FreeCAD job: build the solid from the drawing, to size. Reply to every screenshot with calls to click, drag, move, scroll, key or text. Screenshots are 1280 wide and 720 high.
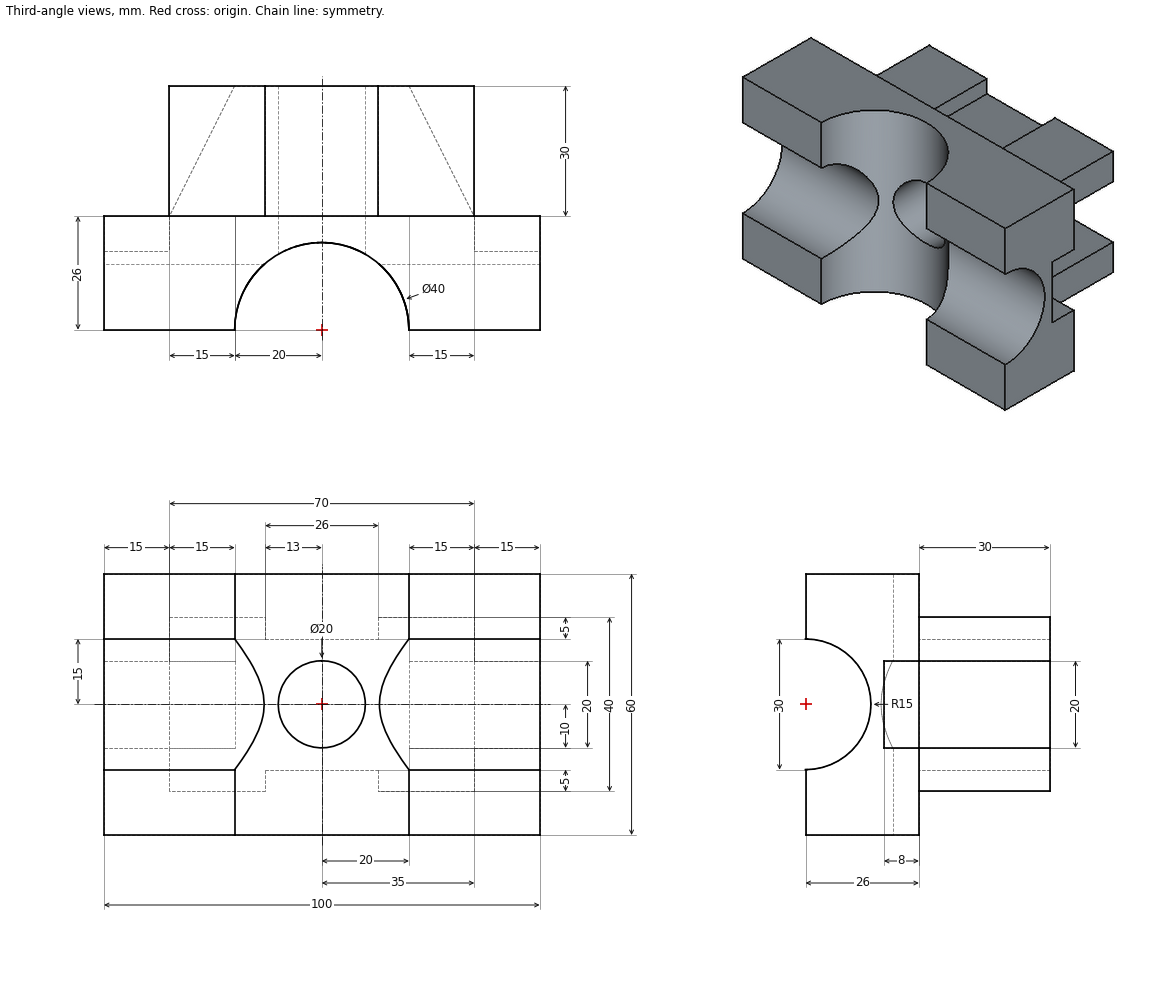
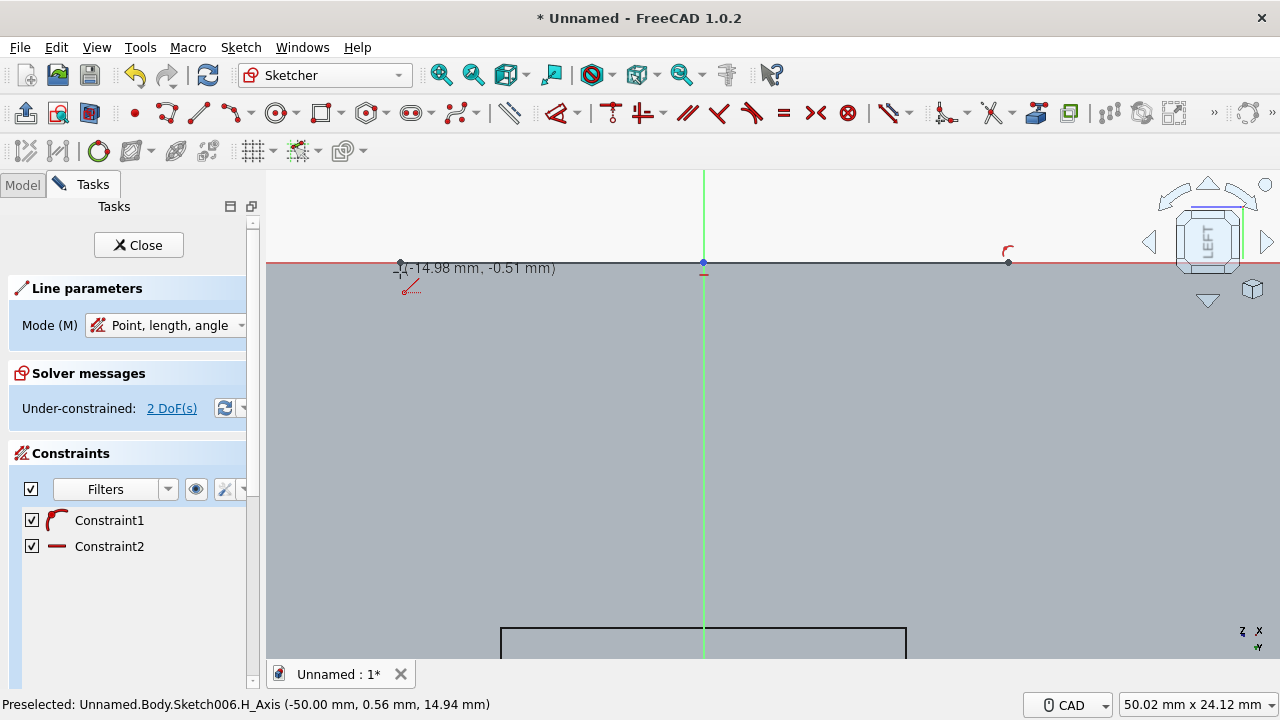
key(g)
key(3)
key(a)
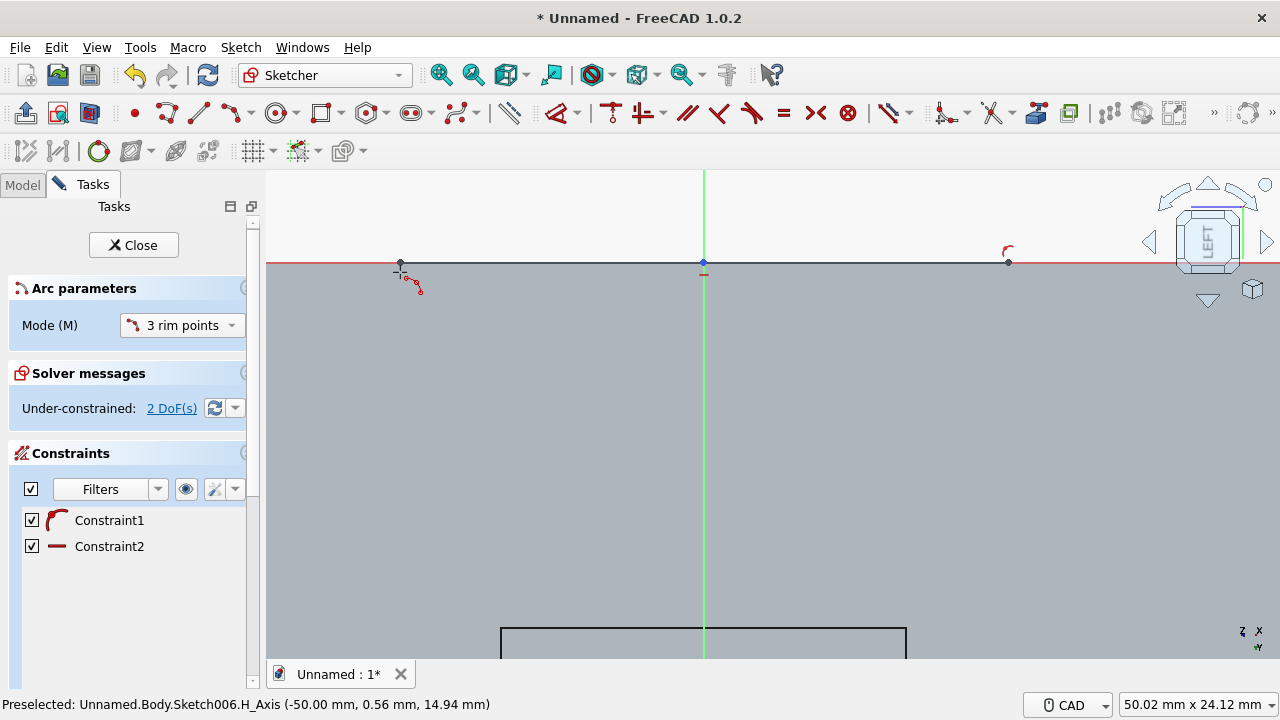
click(400, 272)
click(1008, 263)
click(610, 552)
key(Escape)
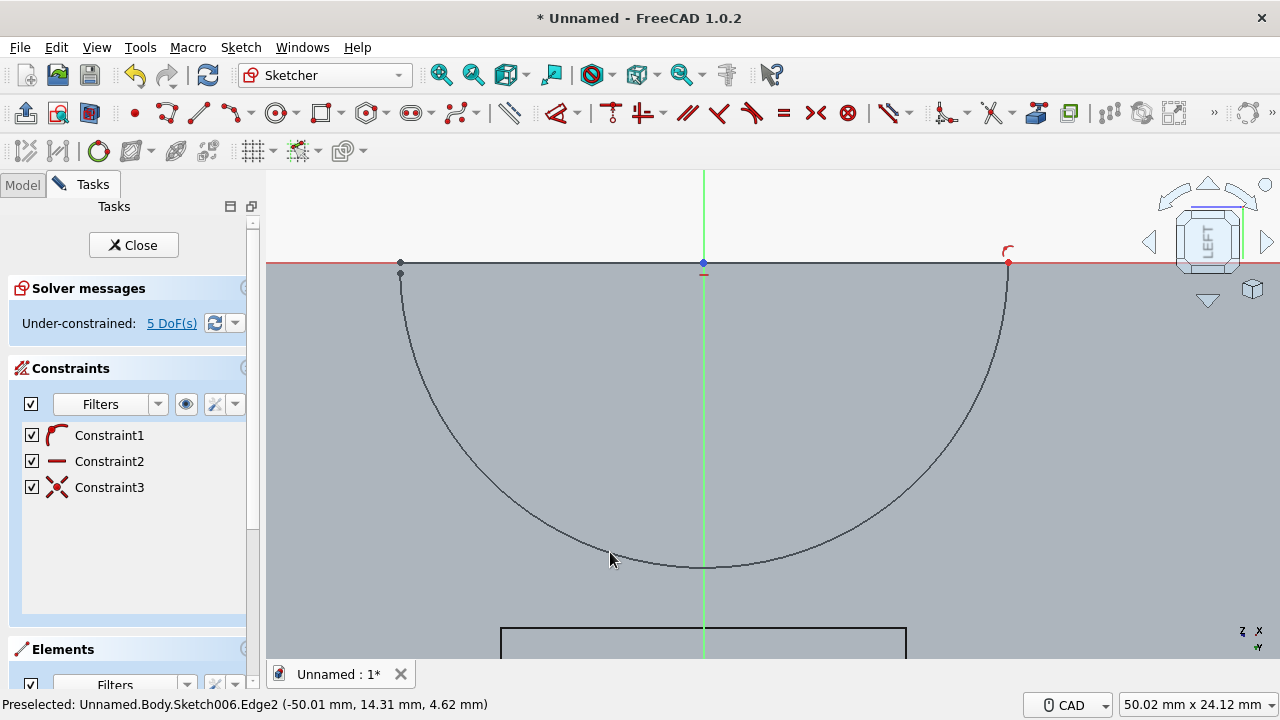
drag(694, 253, 714, 274)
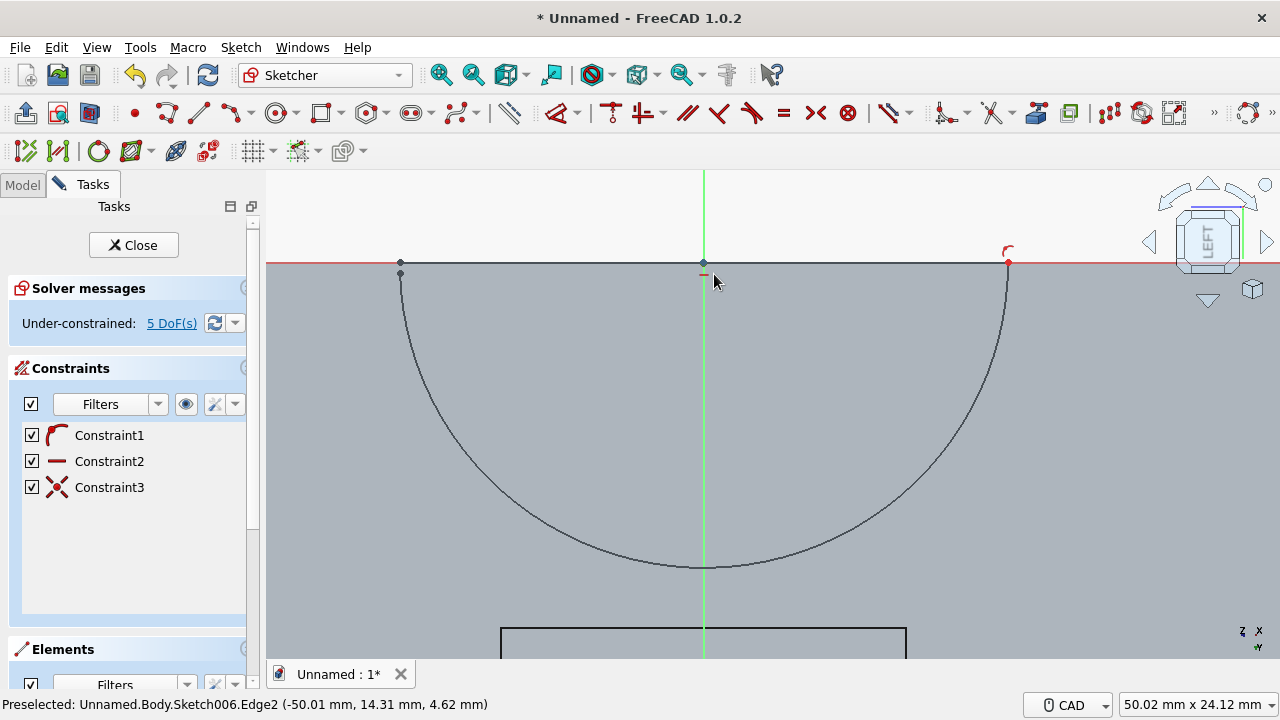
key(c)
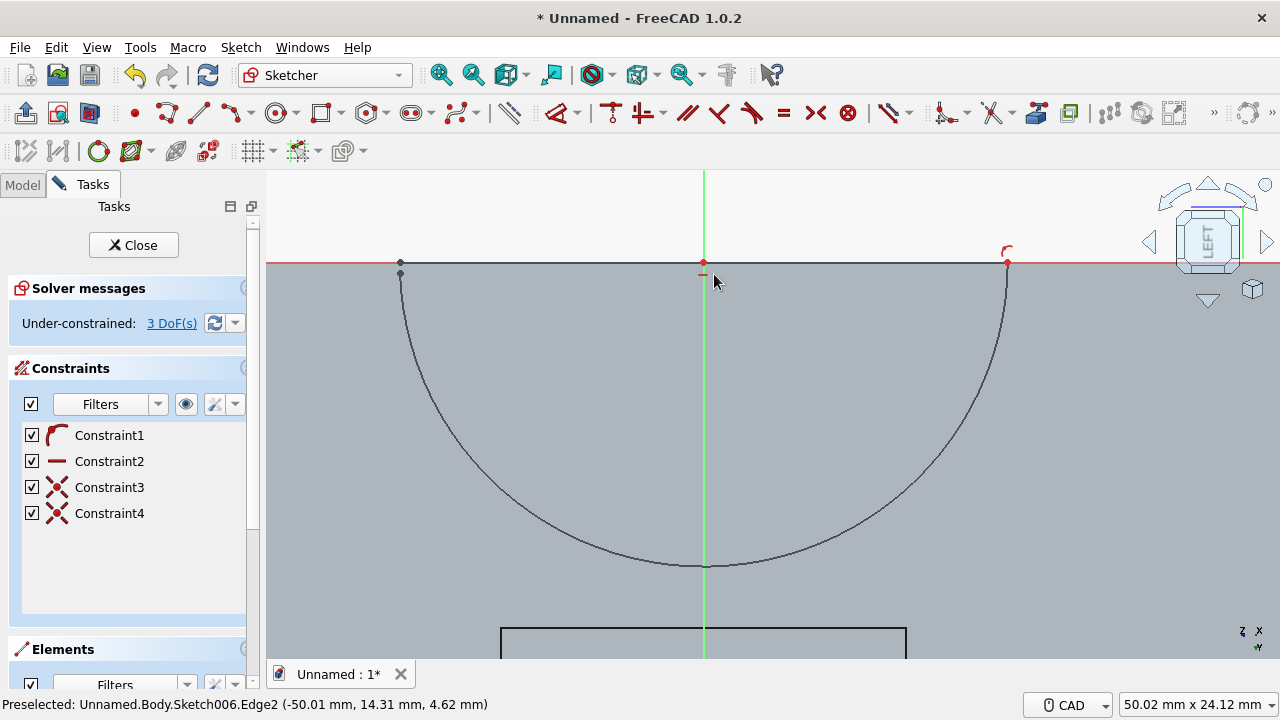
click(556, 114)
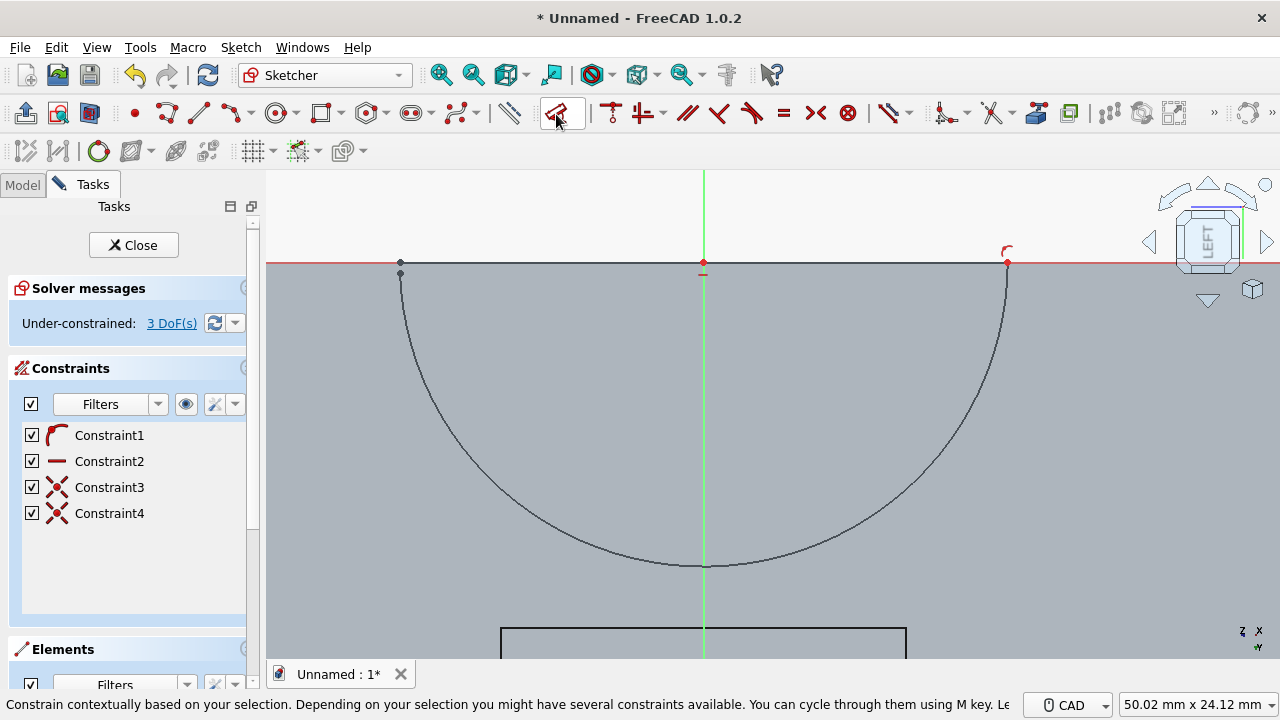
click(531, 513)
click(513, 539)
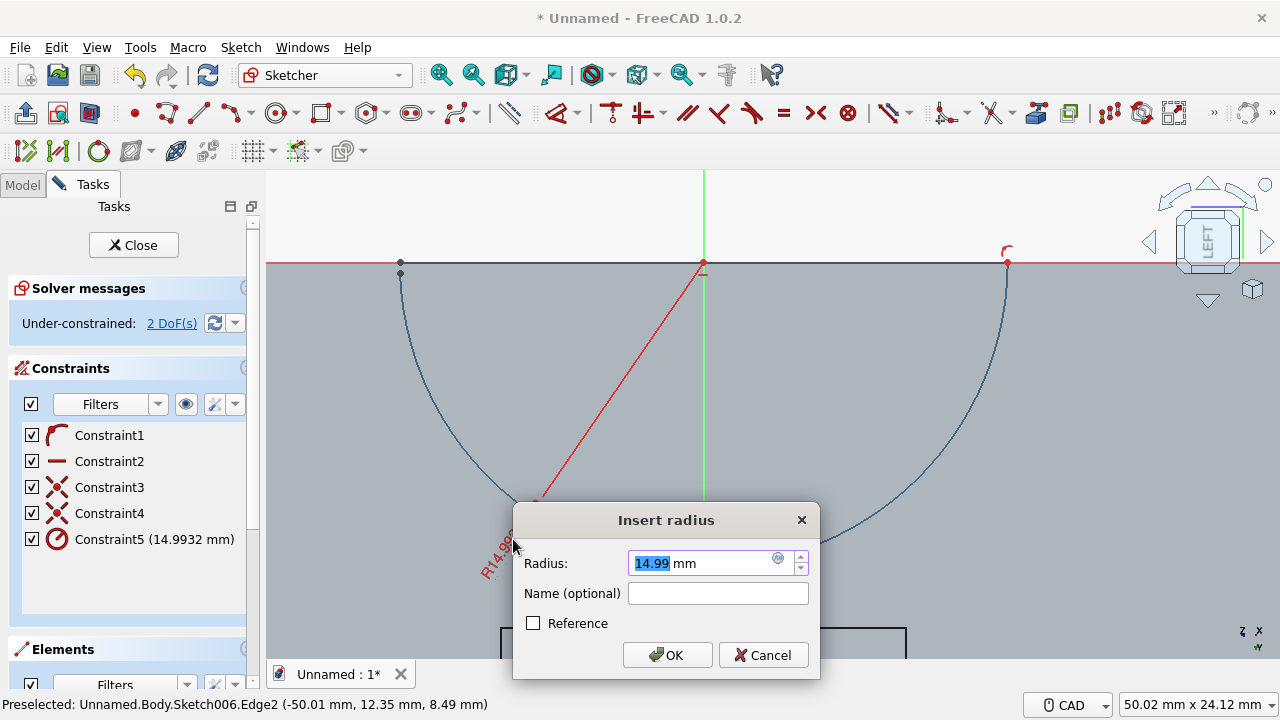
text(15)
key(Return)
key(Escape)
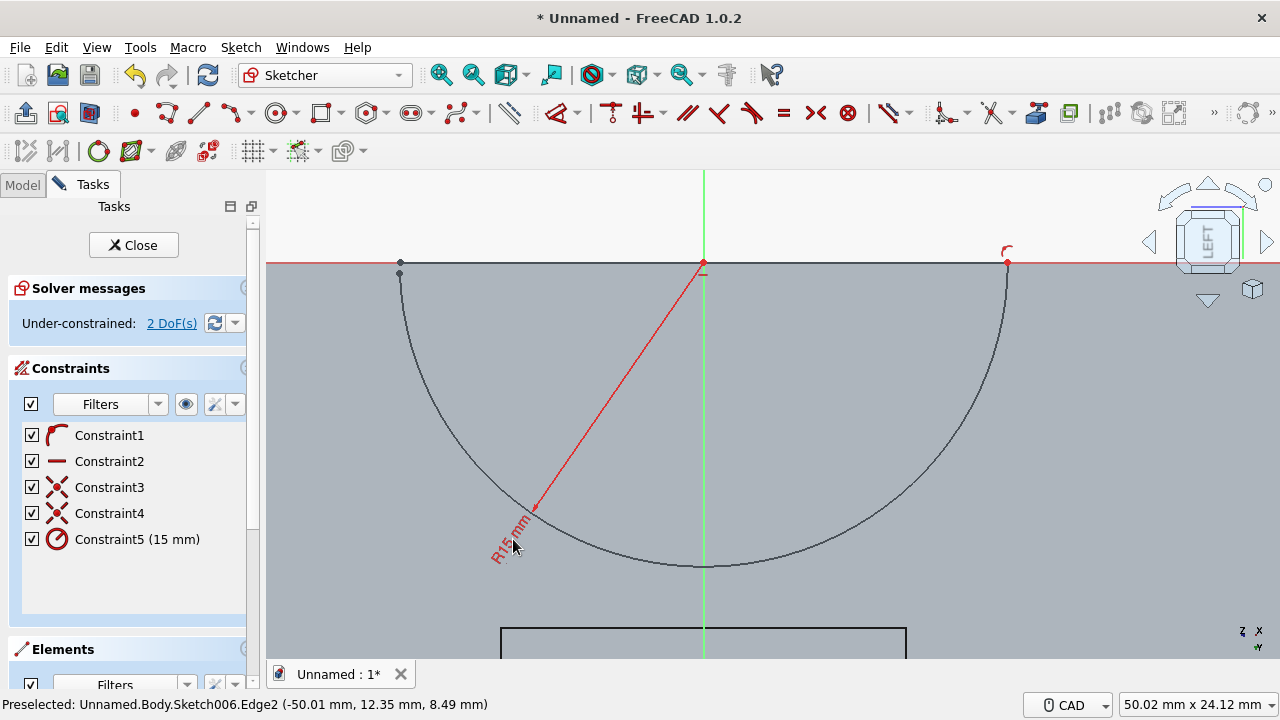
click(400, 273)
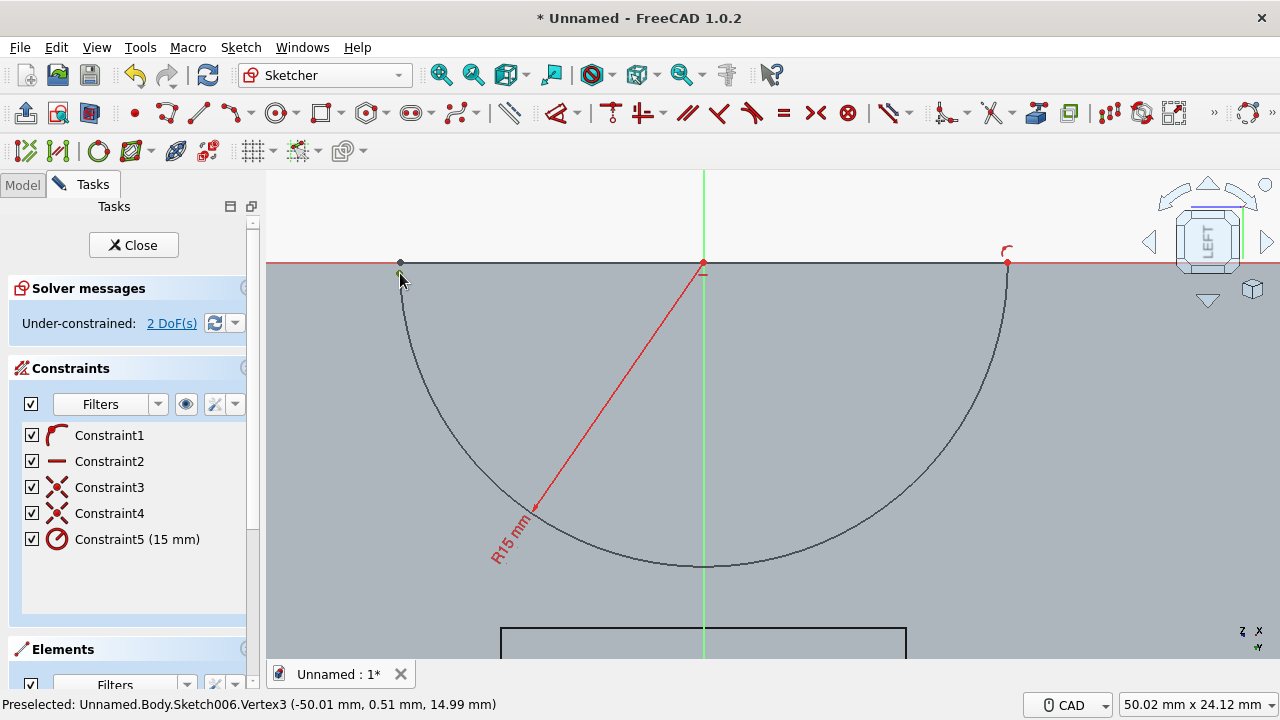
click(353, 263)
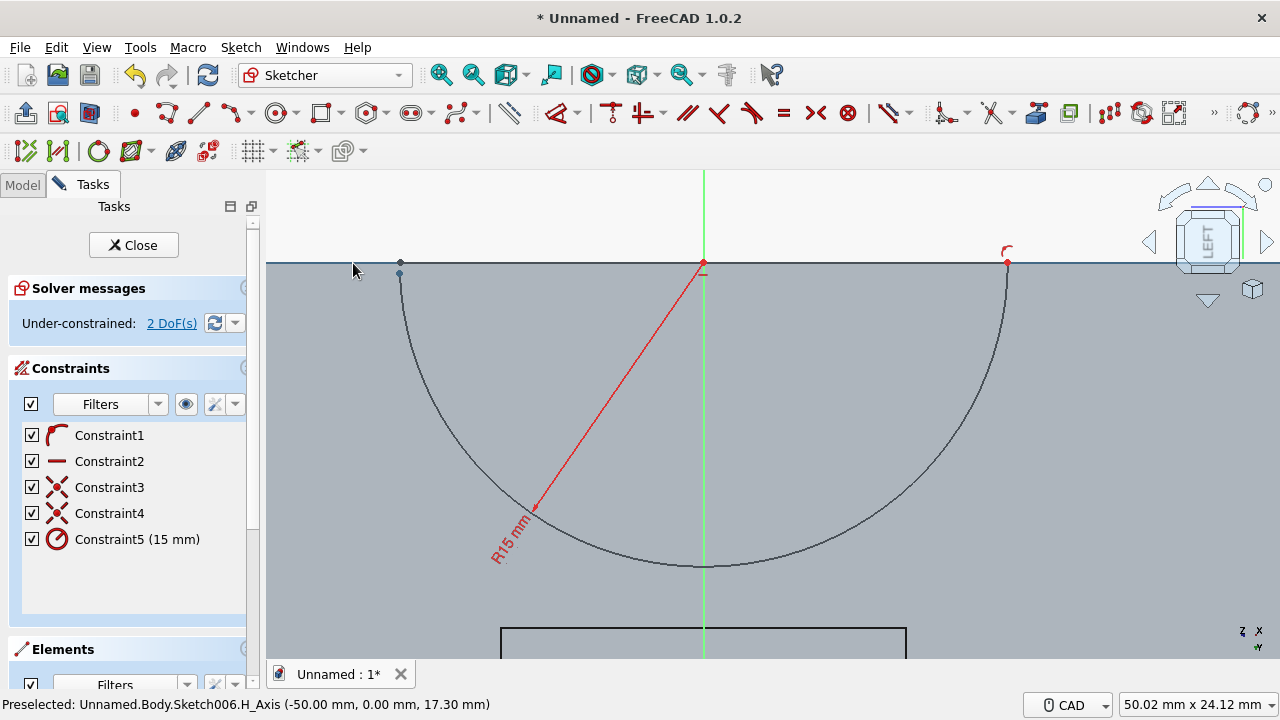
key(c)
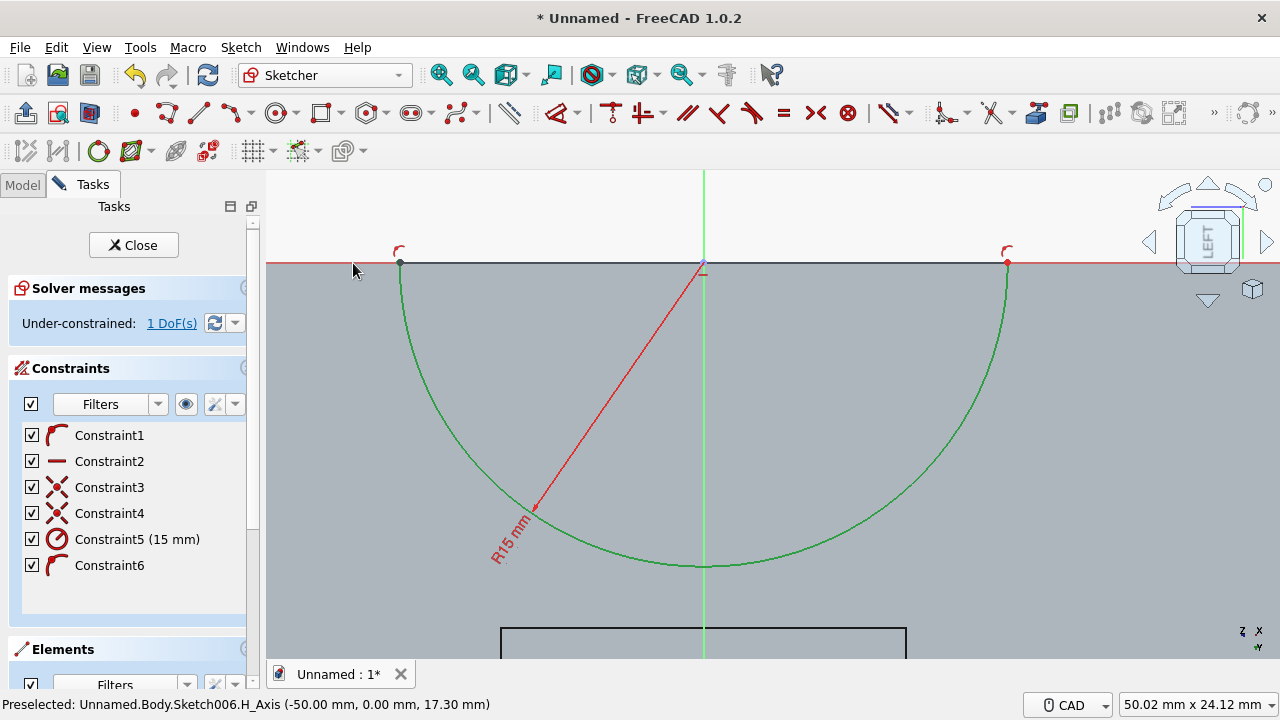
key(d)